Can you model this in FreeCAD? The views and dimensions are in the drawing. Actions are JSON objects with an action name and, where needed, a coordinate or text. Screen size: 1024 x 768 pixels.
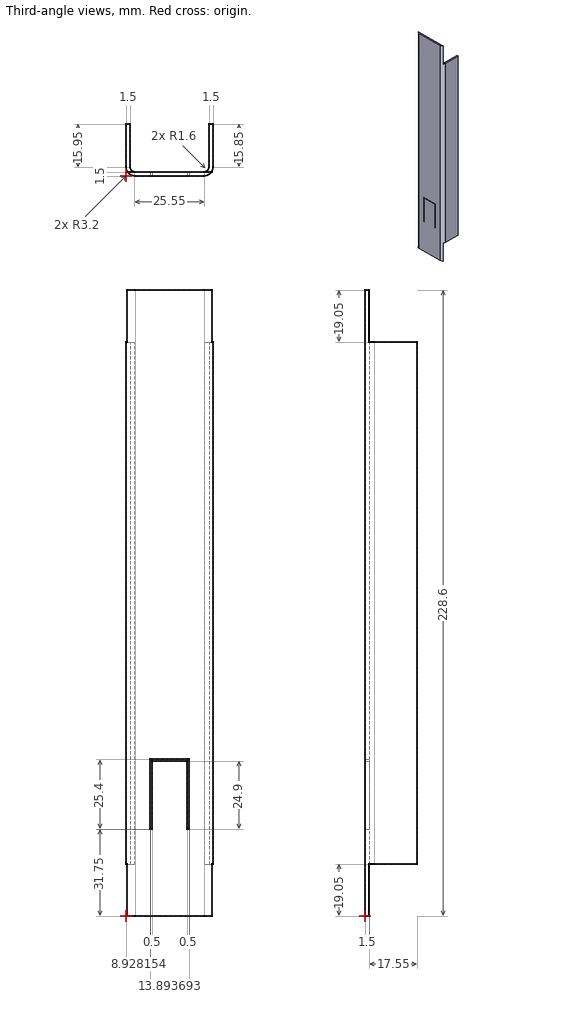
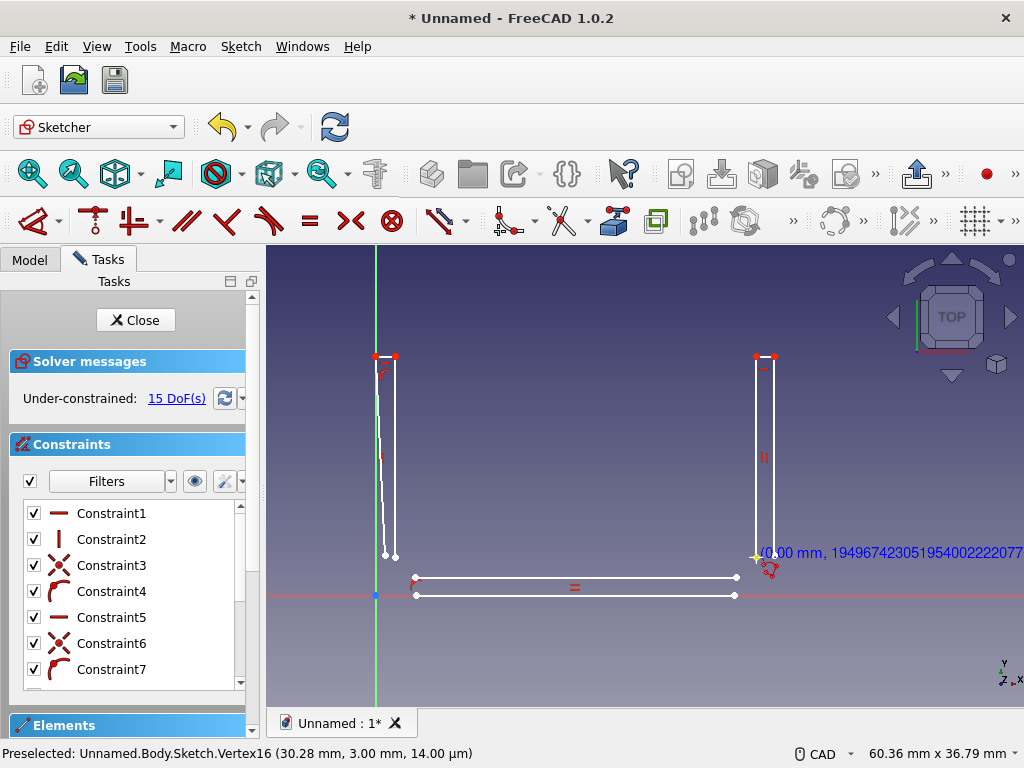
{"action": "key", "text": "g 3 a"}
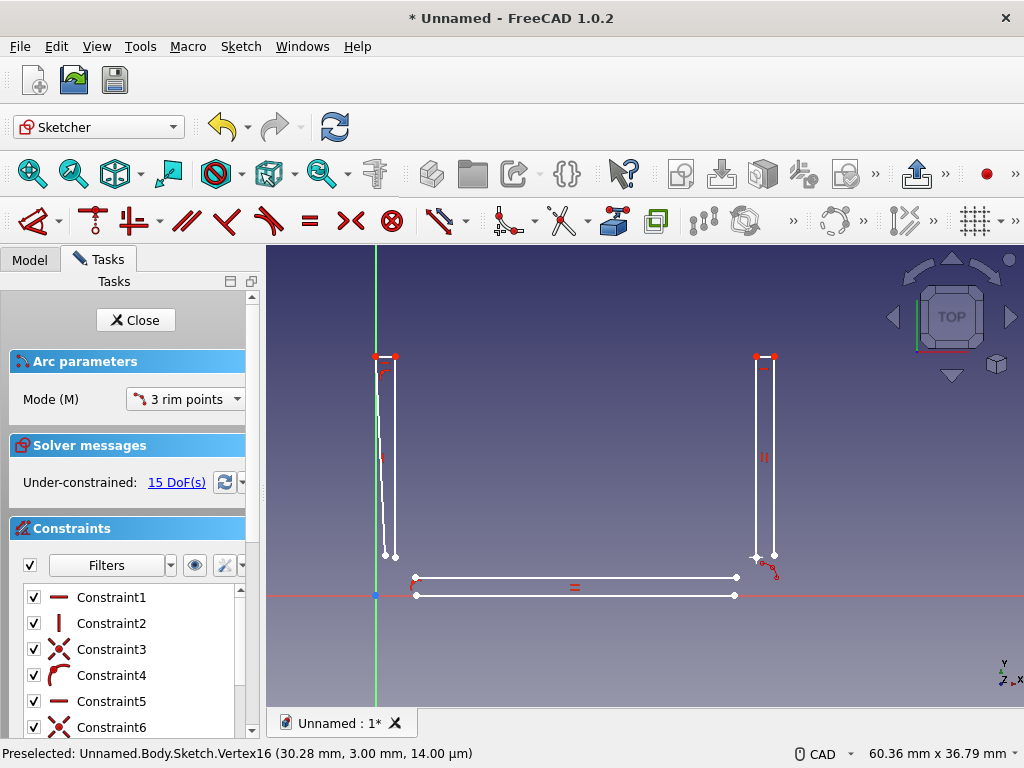
{"action": "left_click", "coordinate": [415, 578]}
{"action": "left_click", "coordinate": [395, 558]}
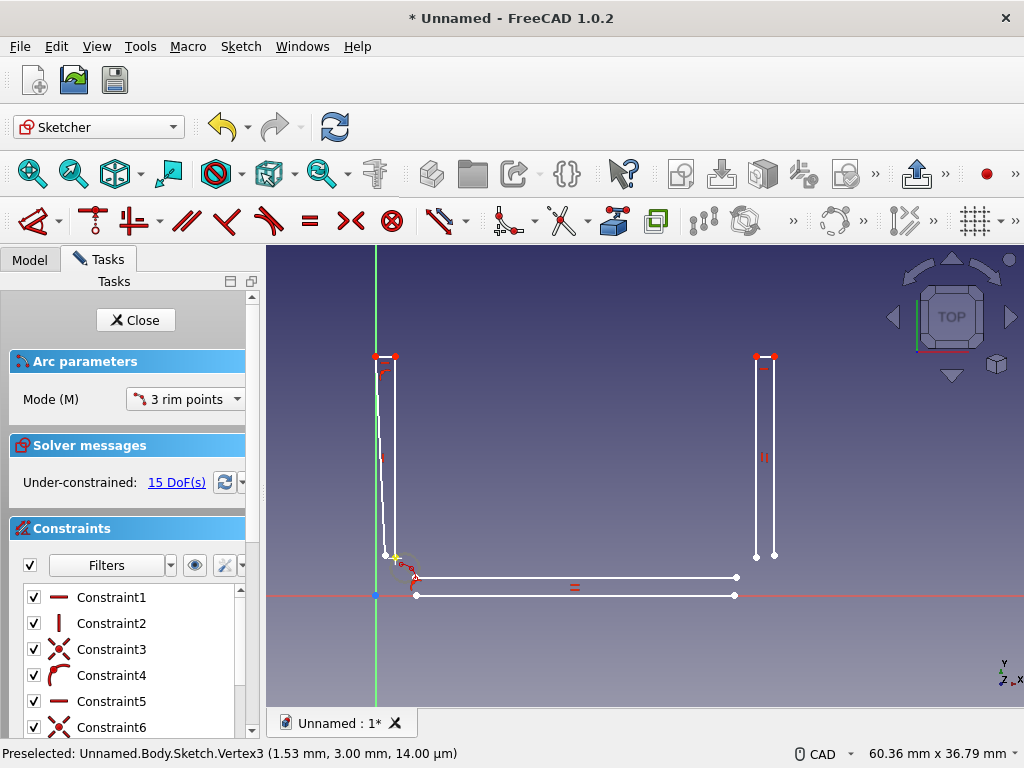
{"action": "scroll", "coordinate": [400, 571], "scroll_direction": "up", "scroll_amount": 5}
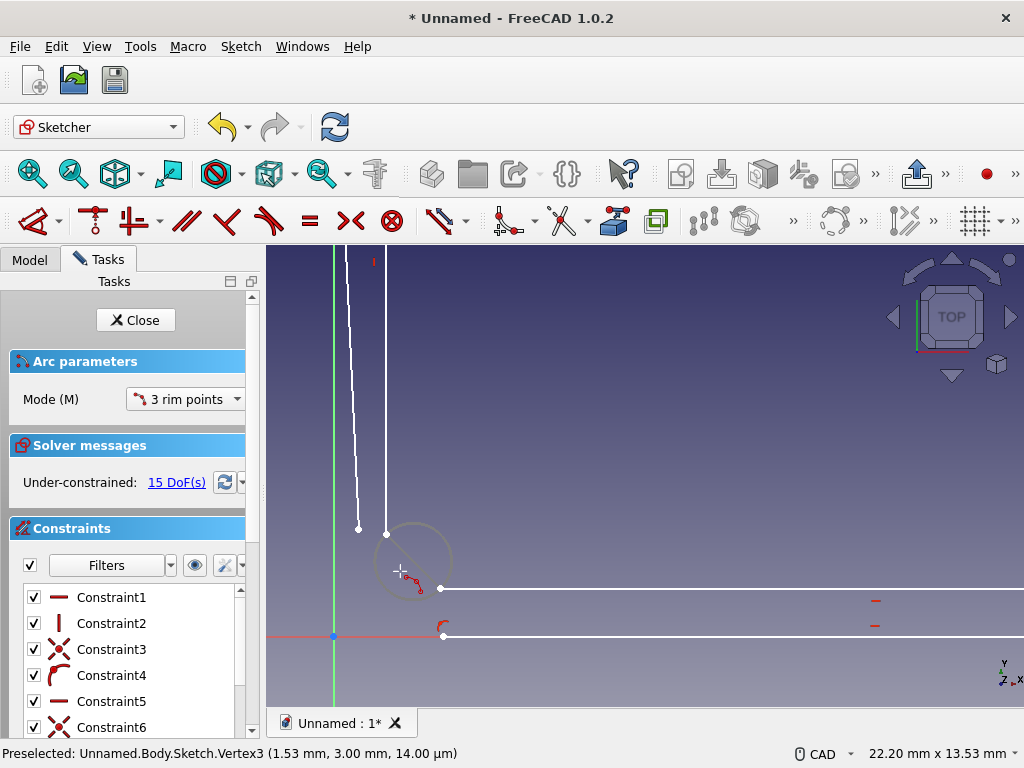
{"action": "left_click", "coordinate": [401, 570]}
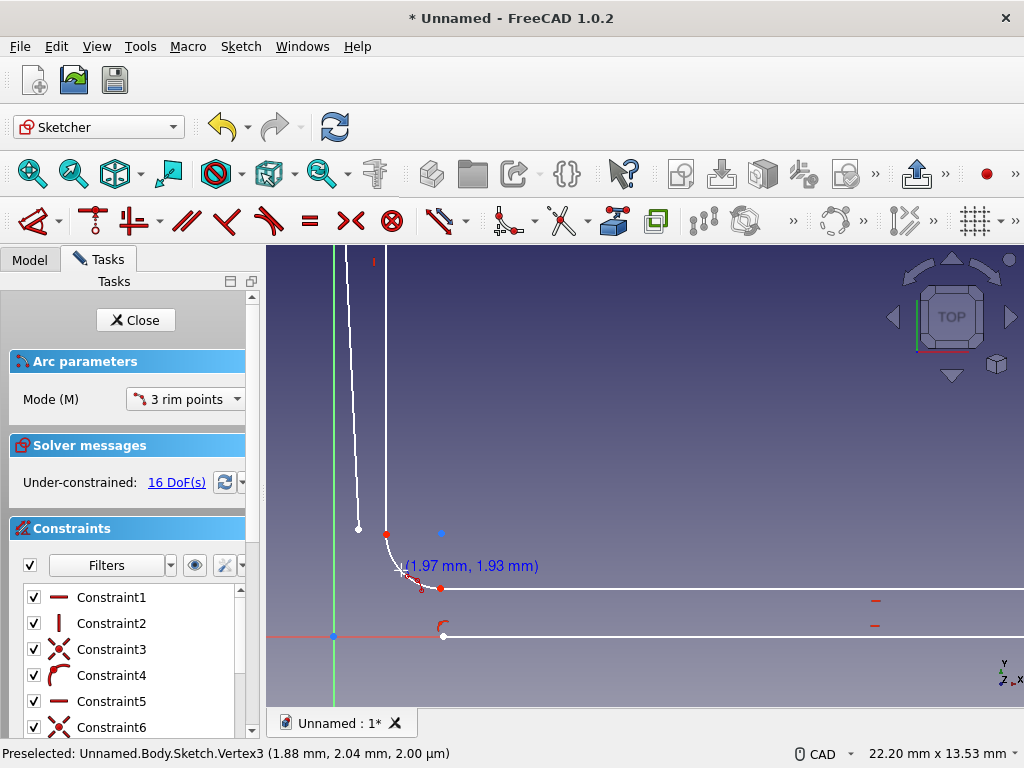
{"action": "left_click", "coordinate": [359, 529]}
{"action": "left_click", "coordinate": [443, 637]}
{"action": "left_click", "coordinate": [366, 605]}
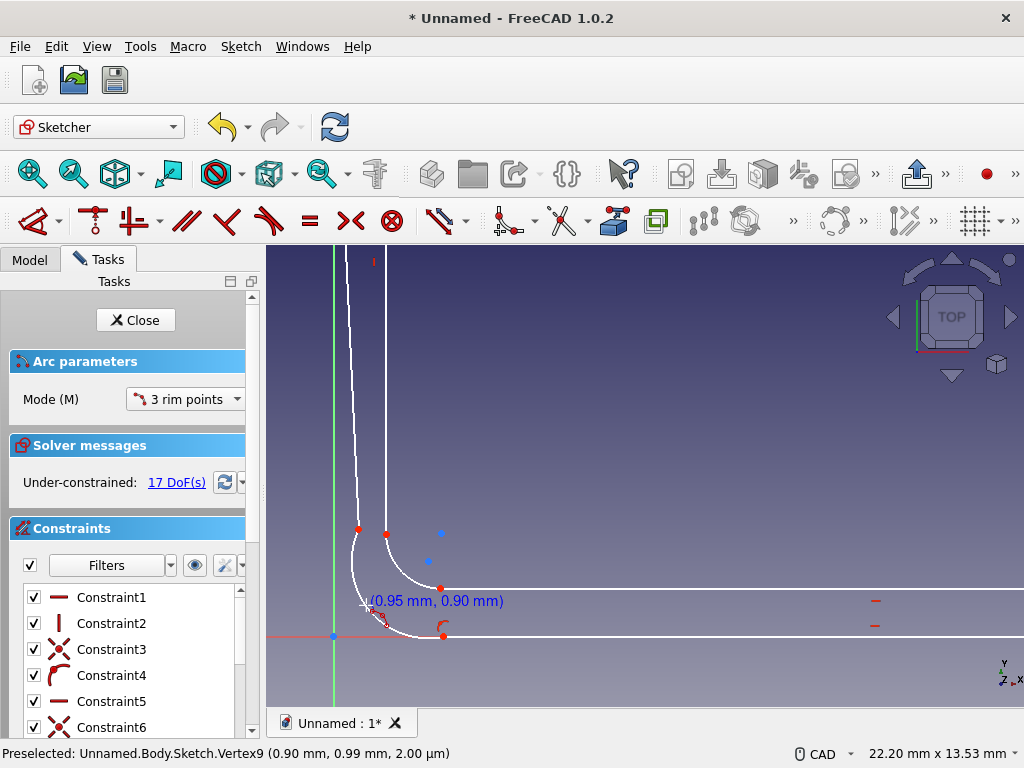
{"action": "scroll", "coordinate": [402, 572], "scroll_direction": "down", "scroll_amount": 5}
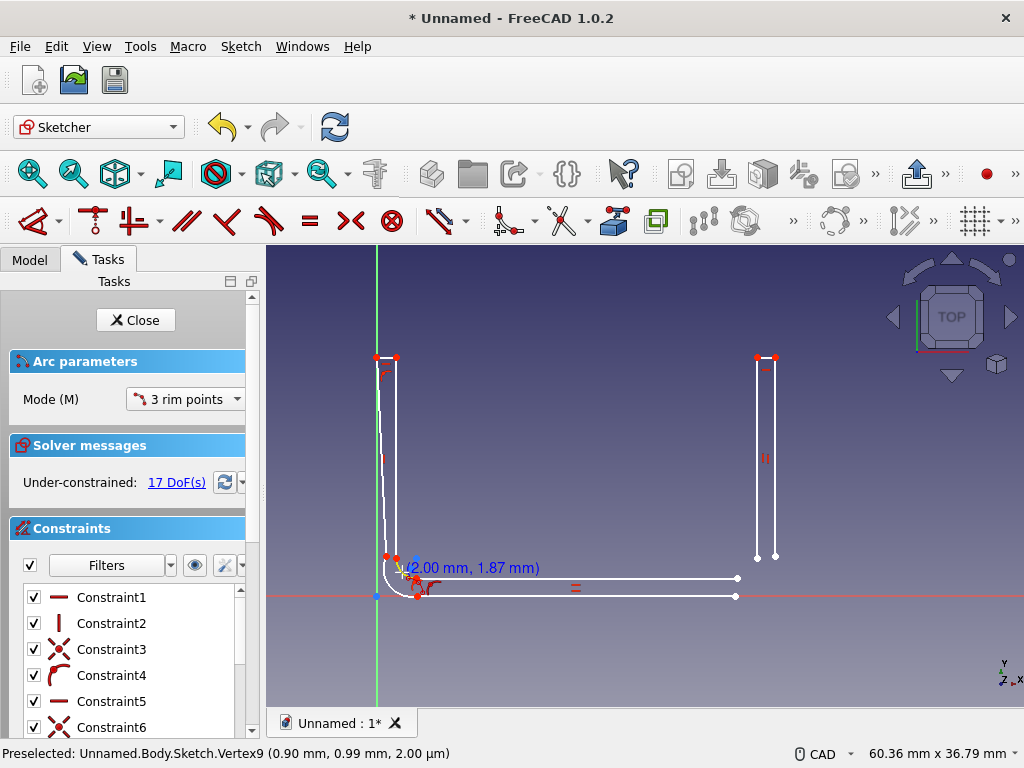
{"action": "left_click", "coordinate": [735, 596]}
{"action": "left_click", "coordinate": [775, 557]}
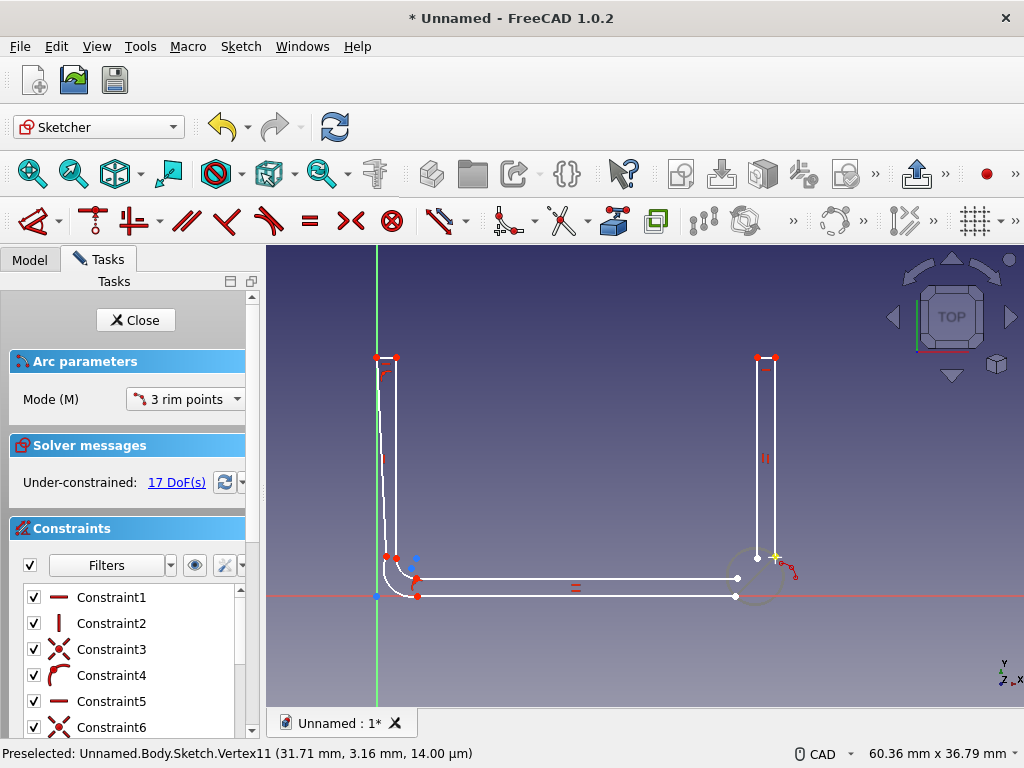
{"action": "scroll", "coordinate": [764, 585], "scroll_direction": "up", "scroll_amount": 2}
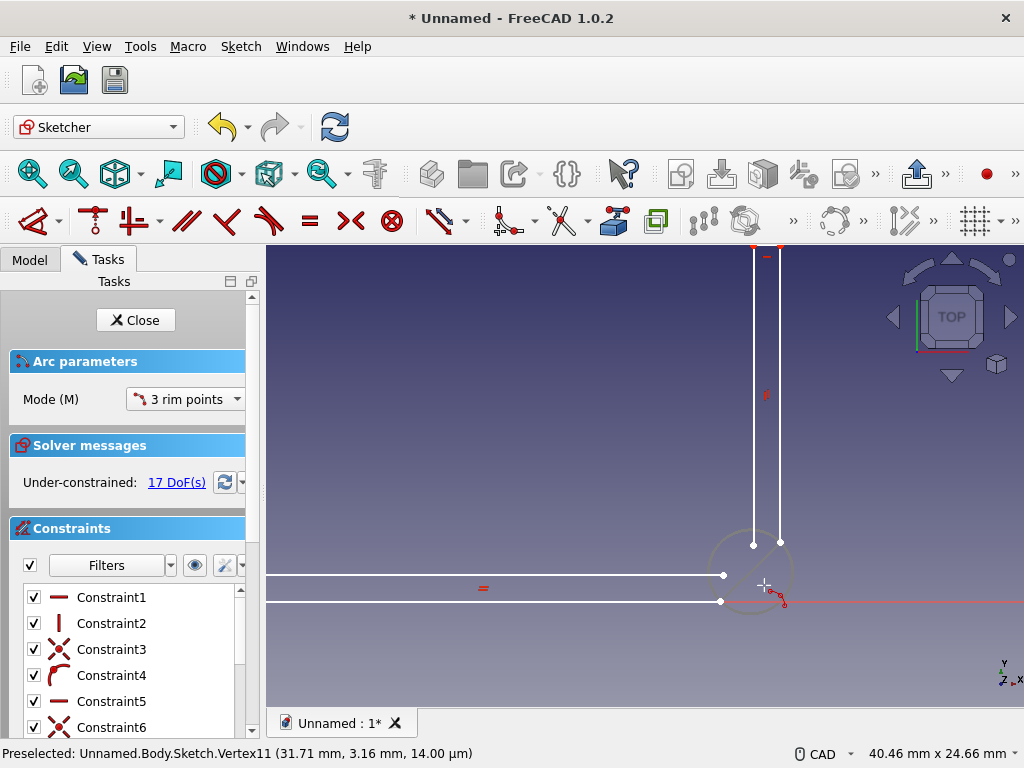
{"action": "left_click", "coordinate": [764, 584]}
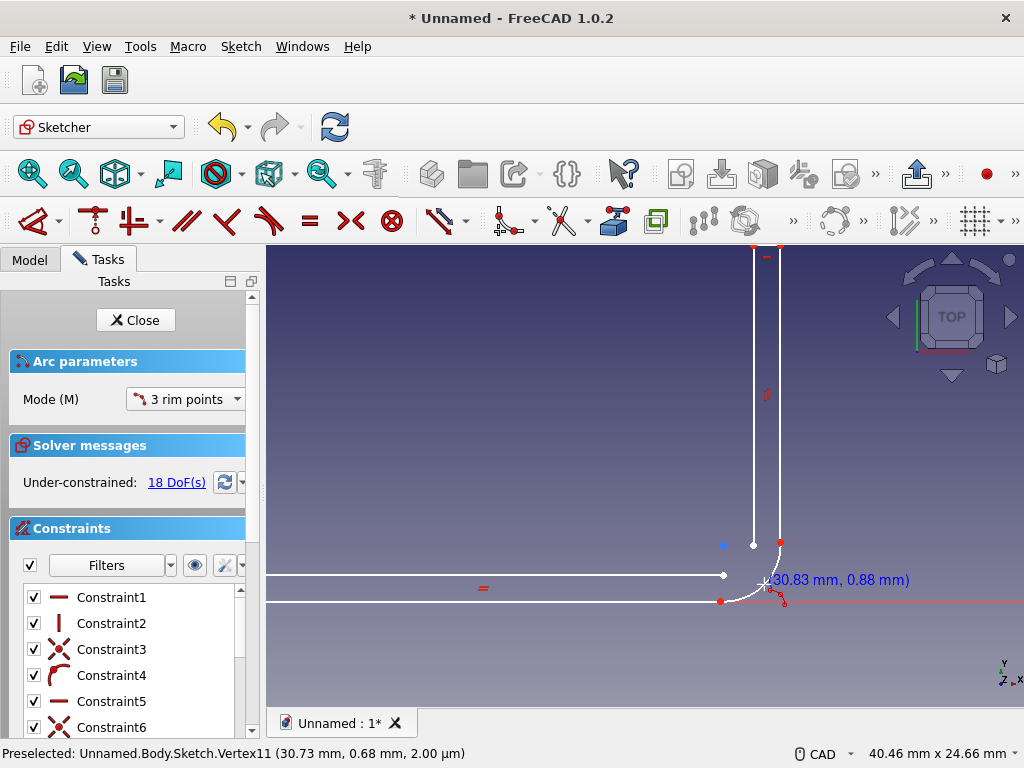
{"action": "left_click", "coordinate": [754, 545]}
{"action": "left_click", "coordinate": [724, 575]}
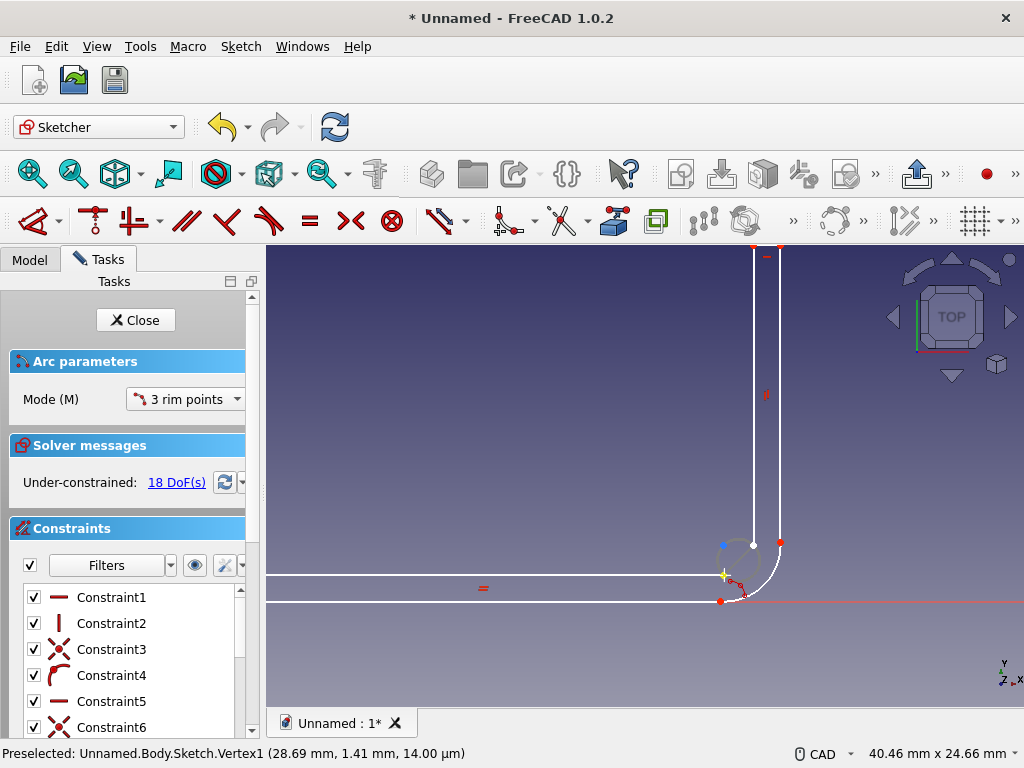
{"action": "scroll", "coordinate": [744, 565], "scroll_direction": "up", "scroll_amount": 3}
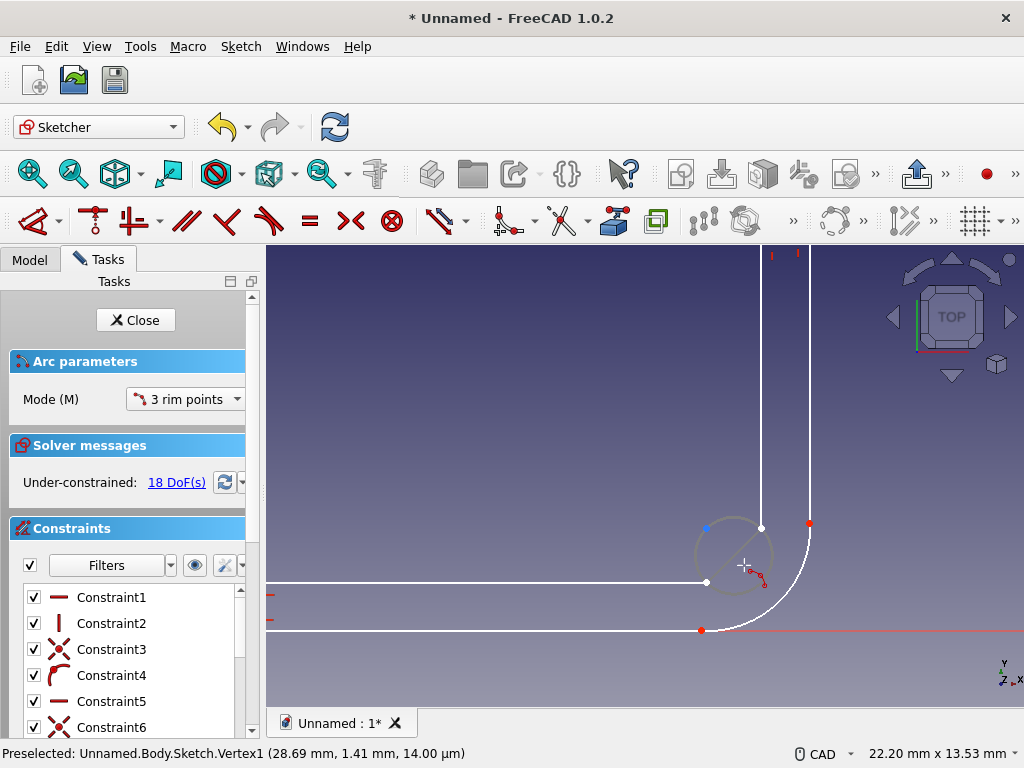
{"action": "left_click", "coordinate": [744, 564]}
{"action": "key", "text": "Escape"}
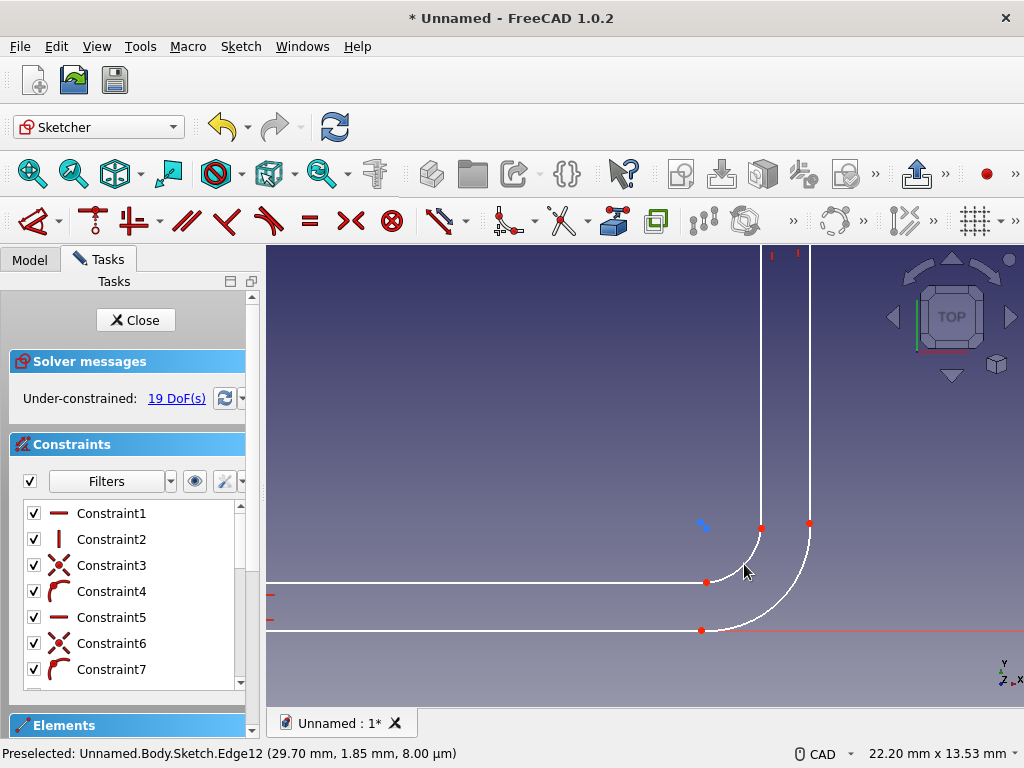
{"action": "left_click", "coordinate": [445, 583]}